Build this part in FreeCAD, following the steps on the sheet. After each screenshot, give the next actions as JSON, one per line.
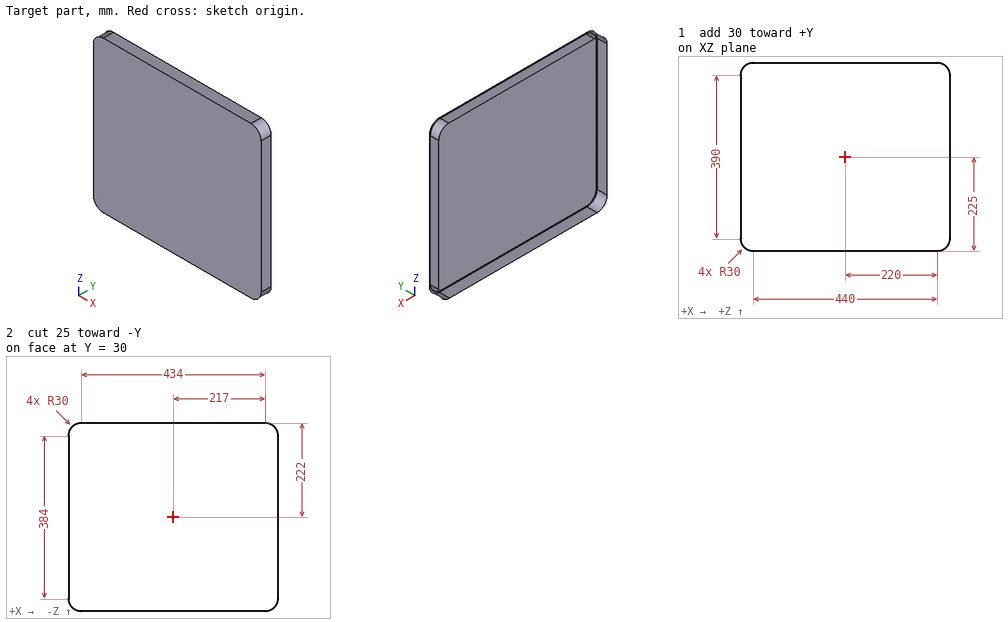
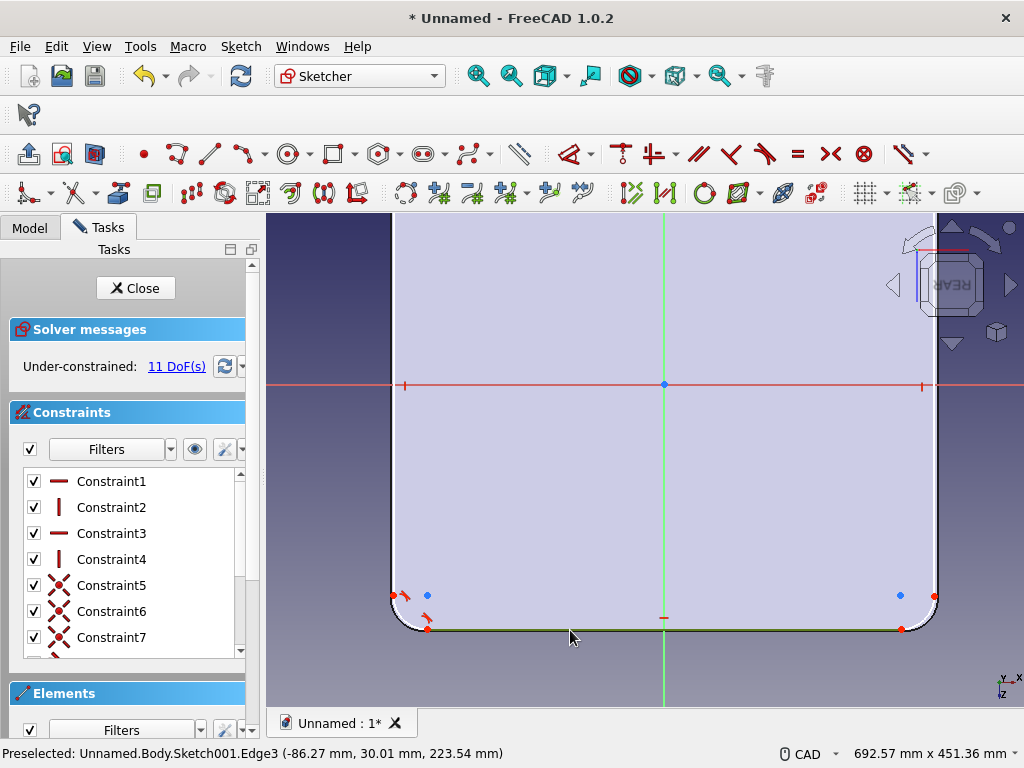
{"action": "scroll", "coordinate": [398, 613], "scroll_direction": "down", "scroll_amount": 2}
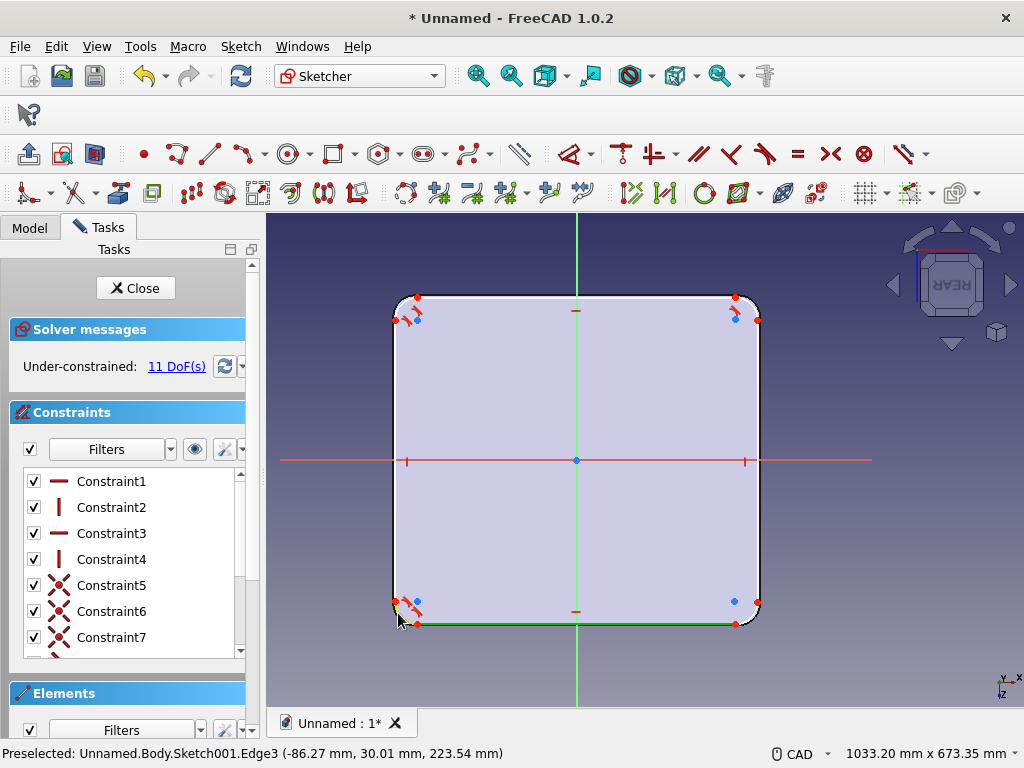
{"action": "scroll", "coordinate": [745, 622], "scroll_direction": "up", "scroll_amount": 2}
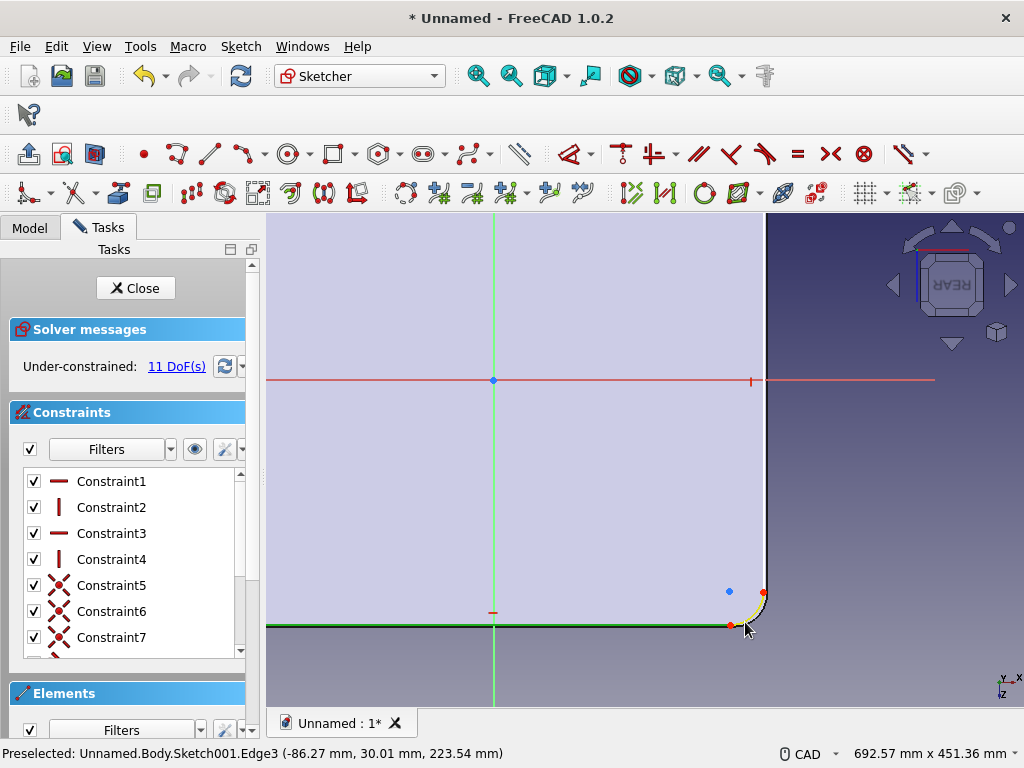
{"action": "left_click", "coordinate": [745, 621]}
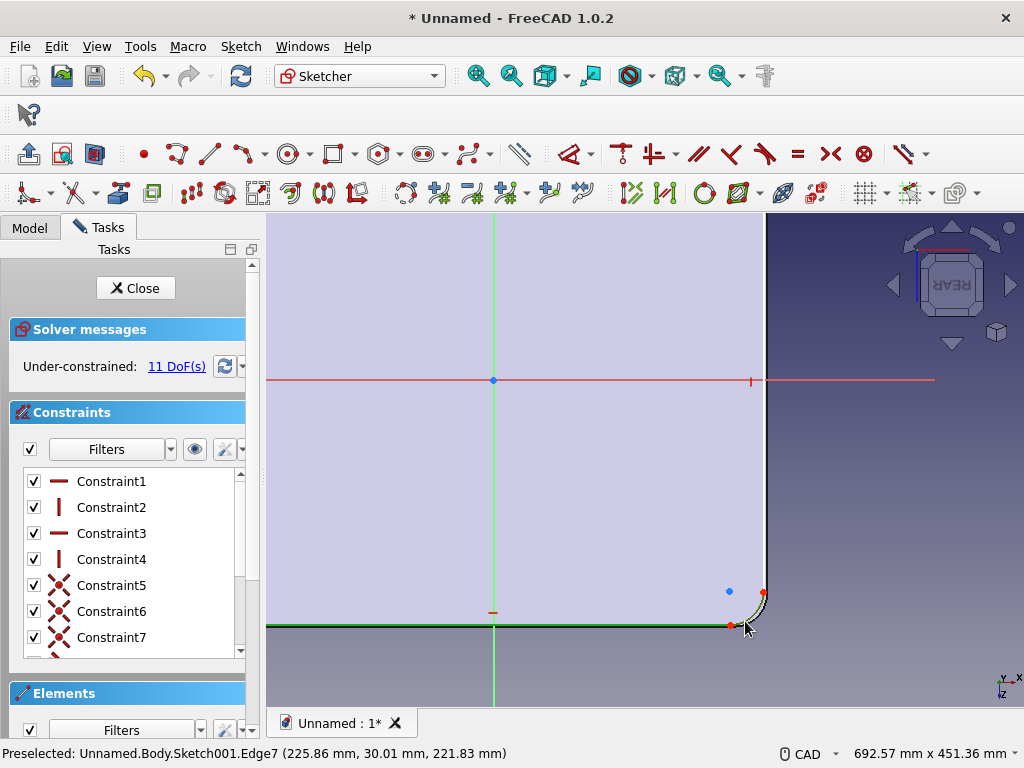
{"action": "left_click", "coordinate": [765, 154]}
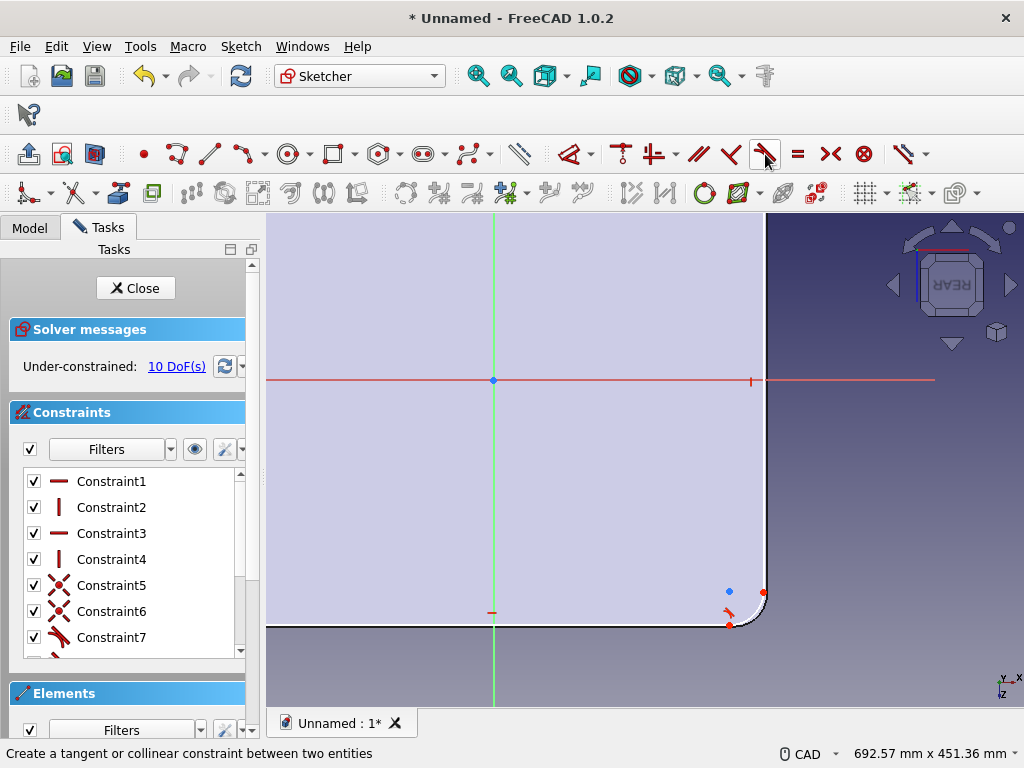
{"action": "left_click", "coordinate": [764, 466]}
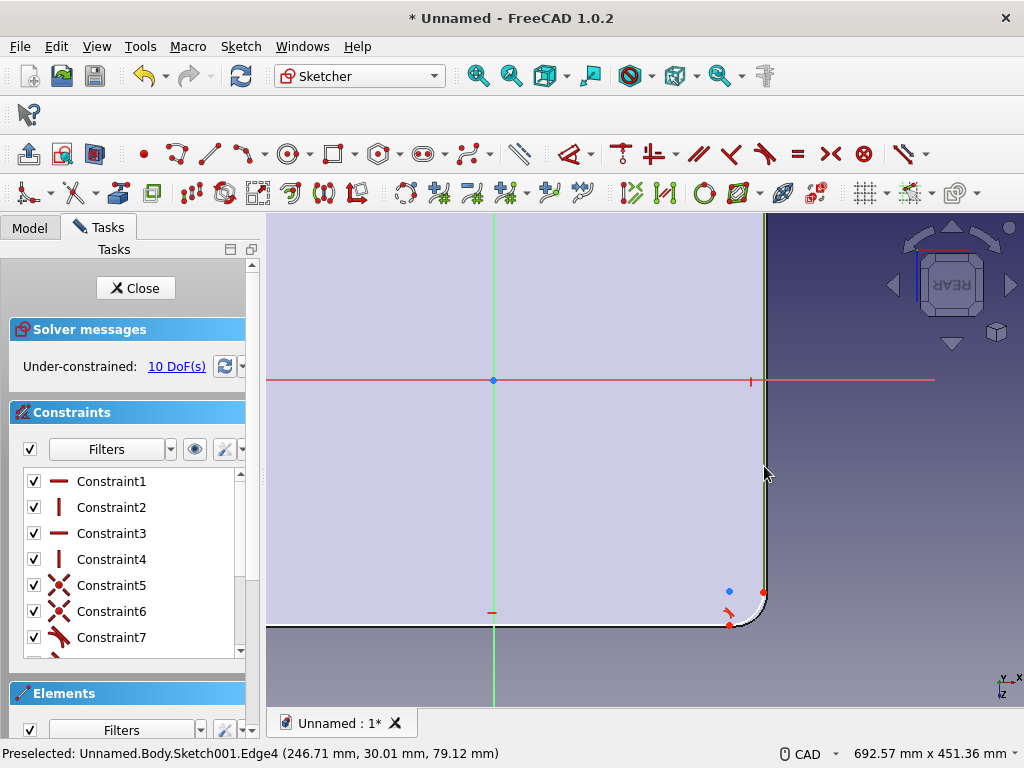
{"action": "left_click", "coordinate": [745, 622]}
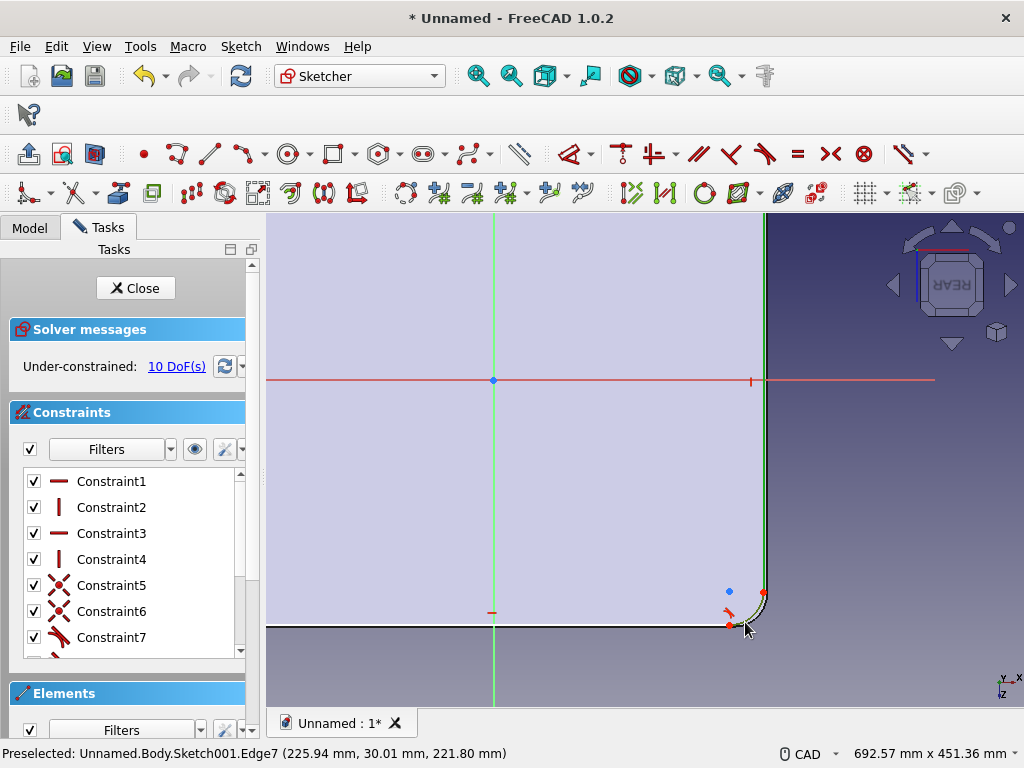
{"action": "left_click", "coordinate": [765, 154]}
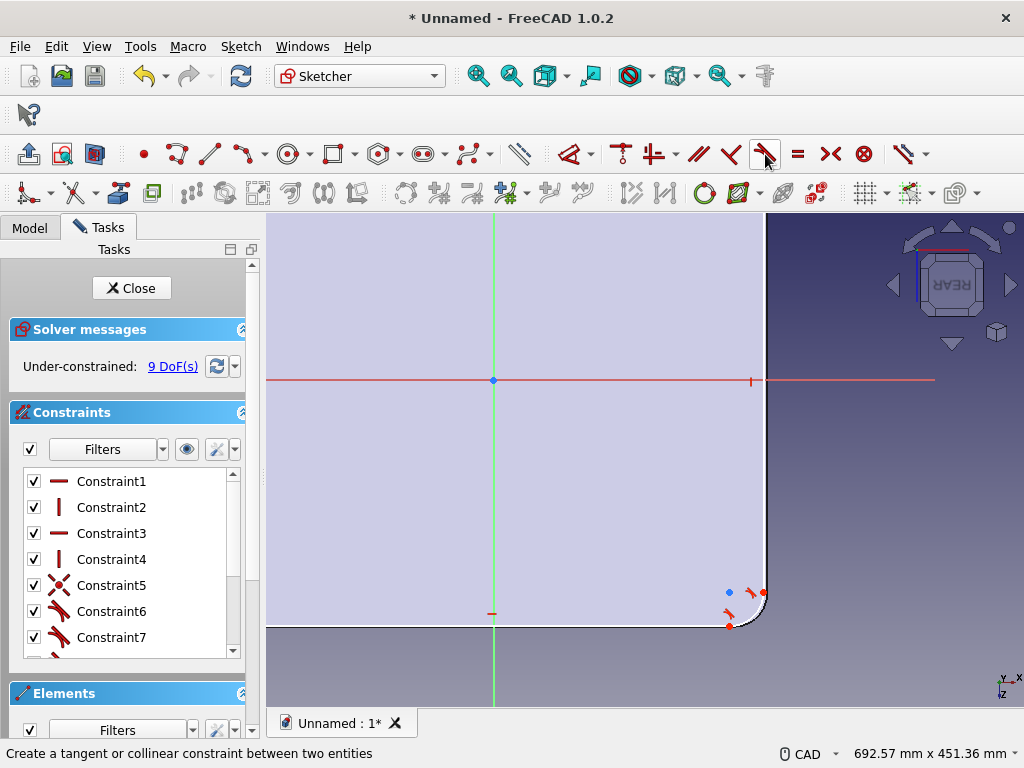
{"action": "left_click", "coordinate": [764, 466]}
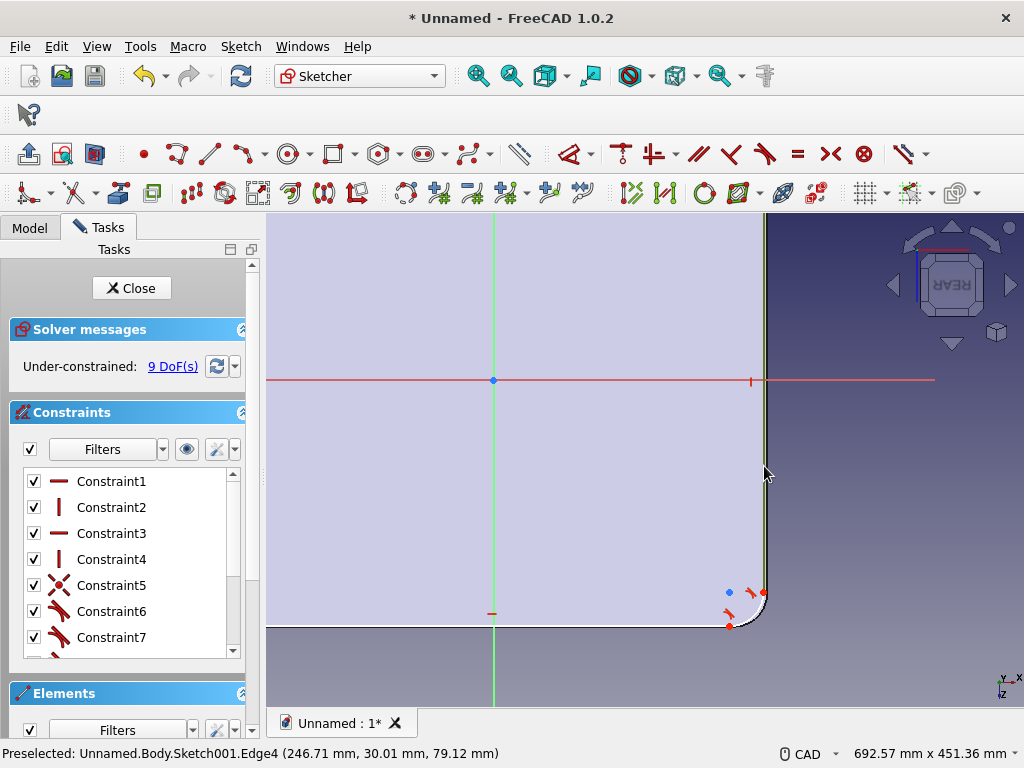
{"action": "scroll", "coordinate": [745, 622], "scroll_direction": "down", "scroll_amount": 2}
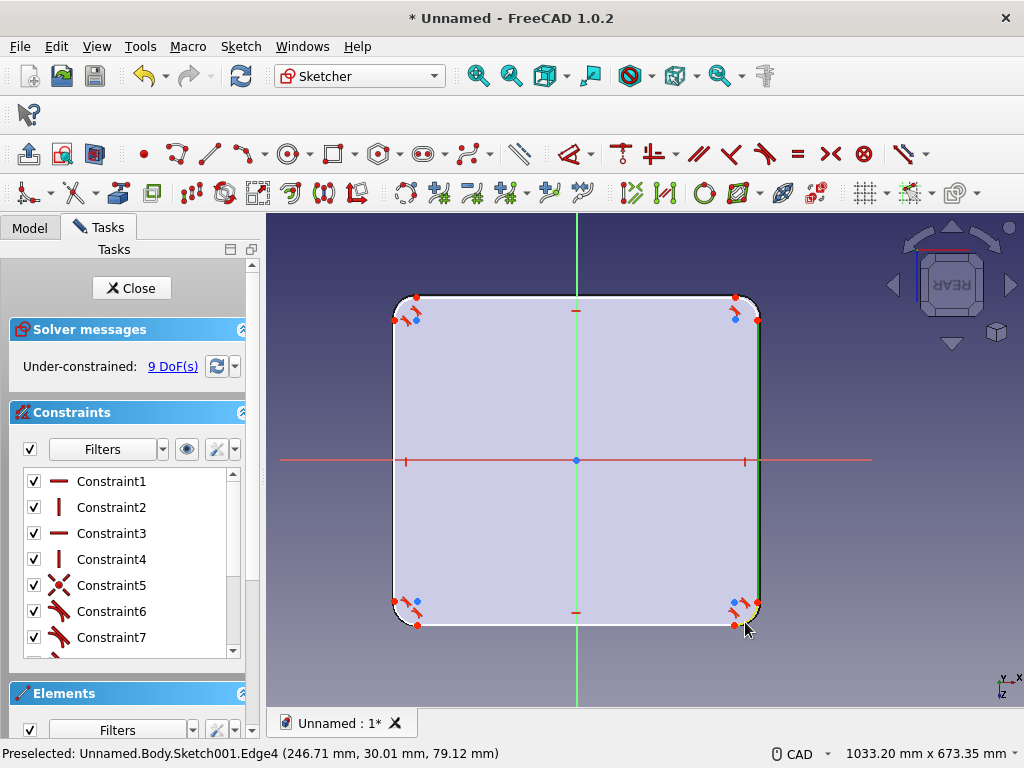
{"action": "scroll", "coordinate": [755, 310], "scroll_direction": "up", "scroll_amount": 2}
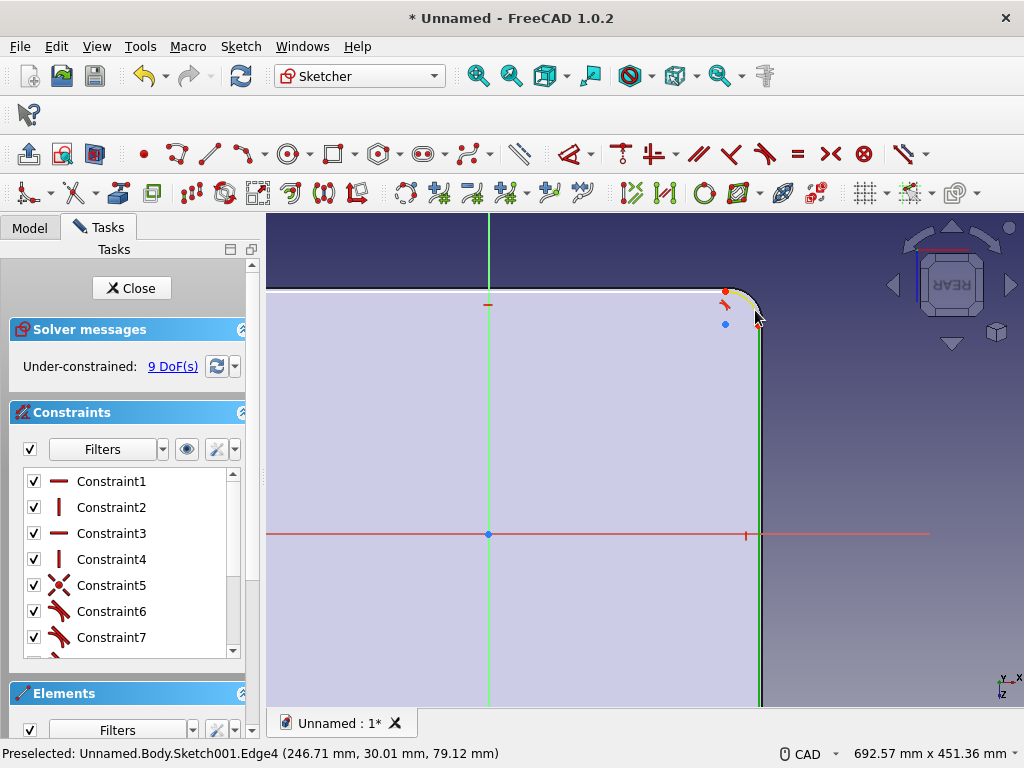
{"action": "left_click", "coordinate": [755, 310]}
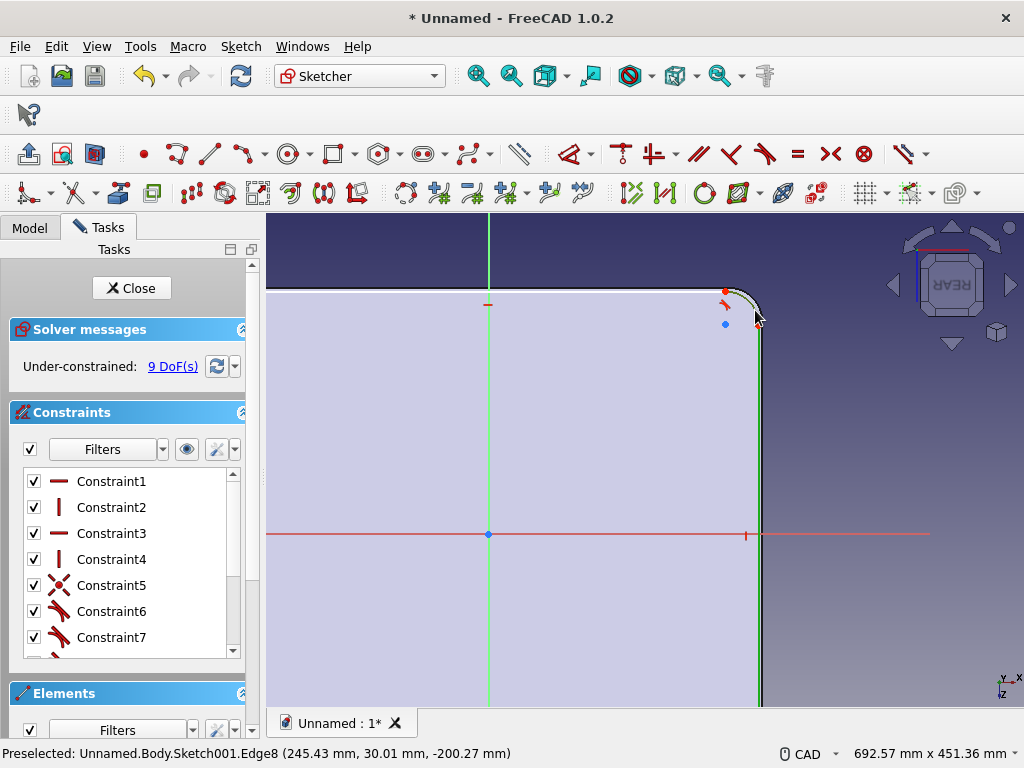
{"action": "left_click", "coordinate": [765, 154]}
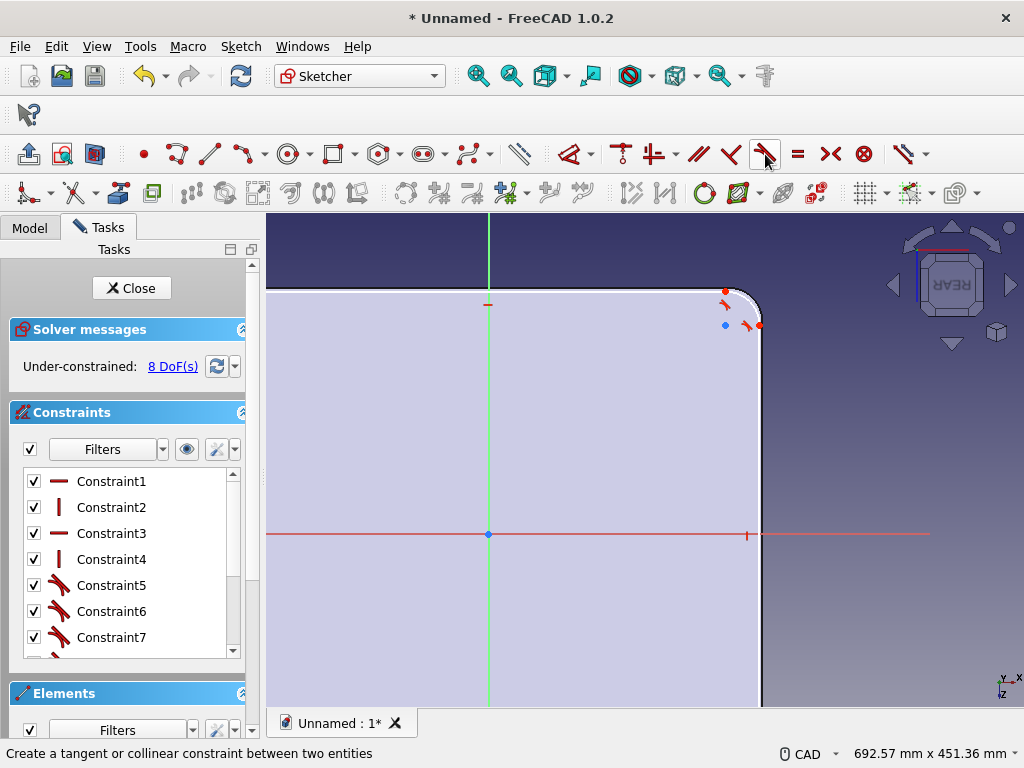
{"action": "scroll", "coordinate": [755, 309], "scroll_direction": "down", "scroll_amount": 2}